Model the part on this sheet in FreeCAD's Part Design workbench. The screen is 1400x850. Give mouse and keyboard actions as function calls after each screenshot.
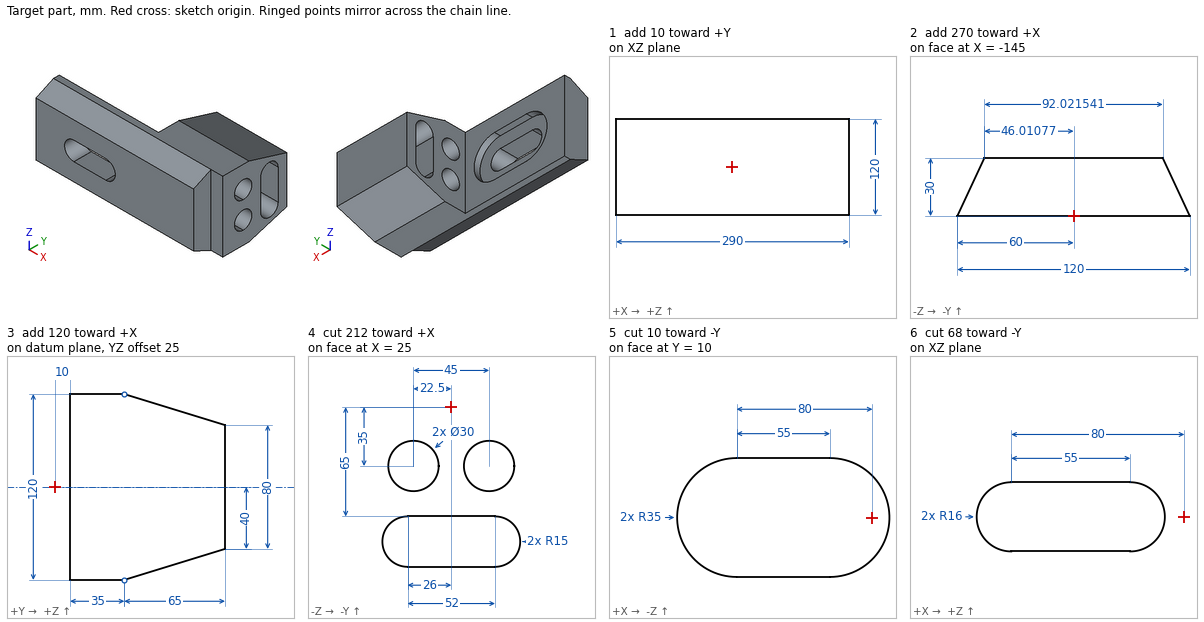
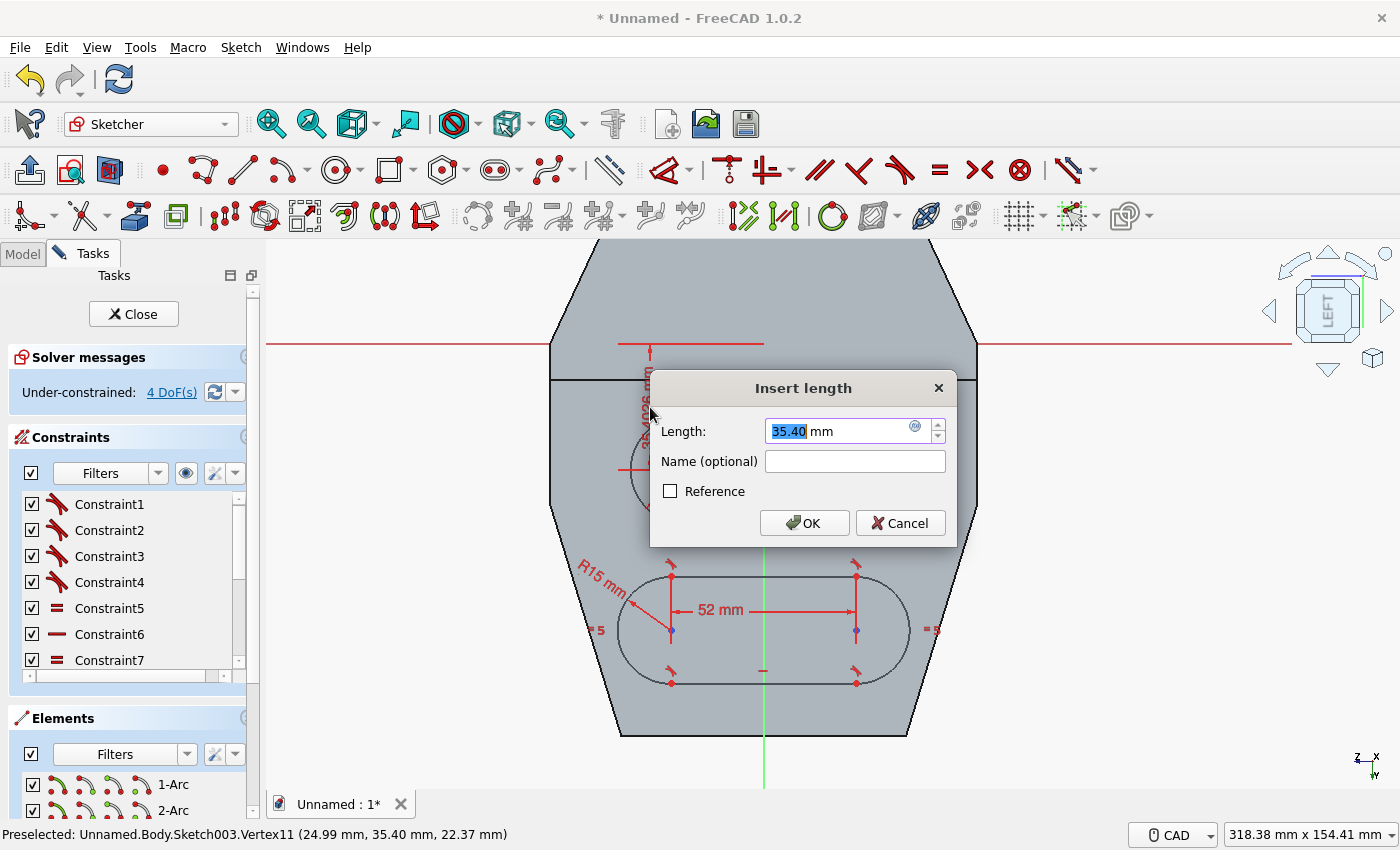
text(35)
key(Return)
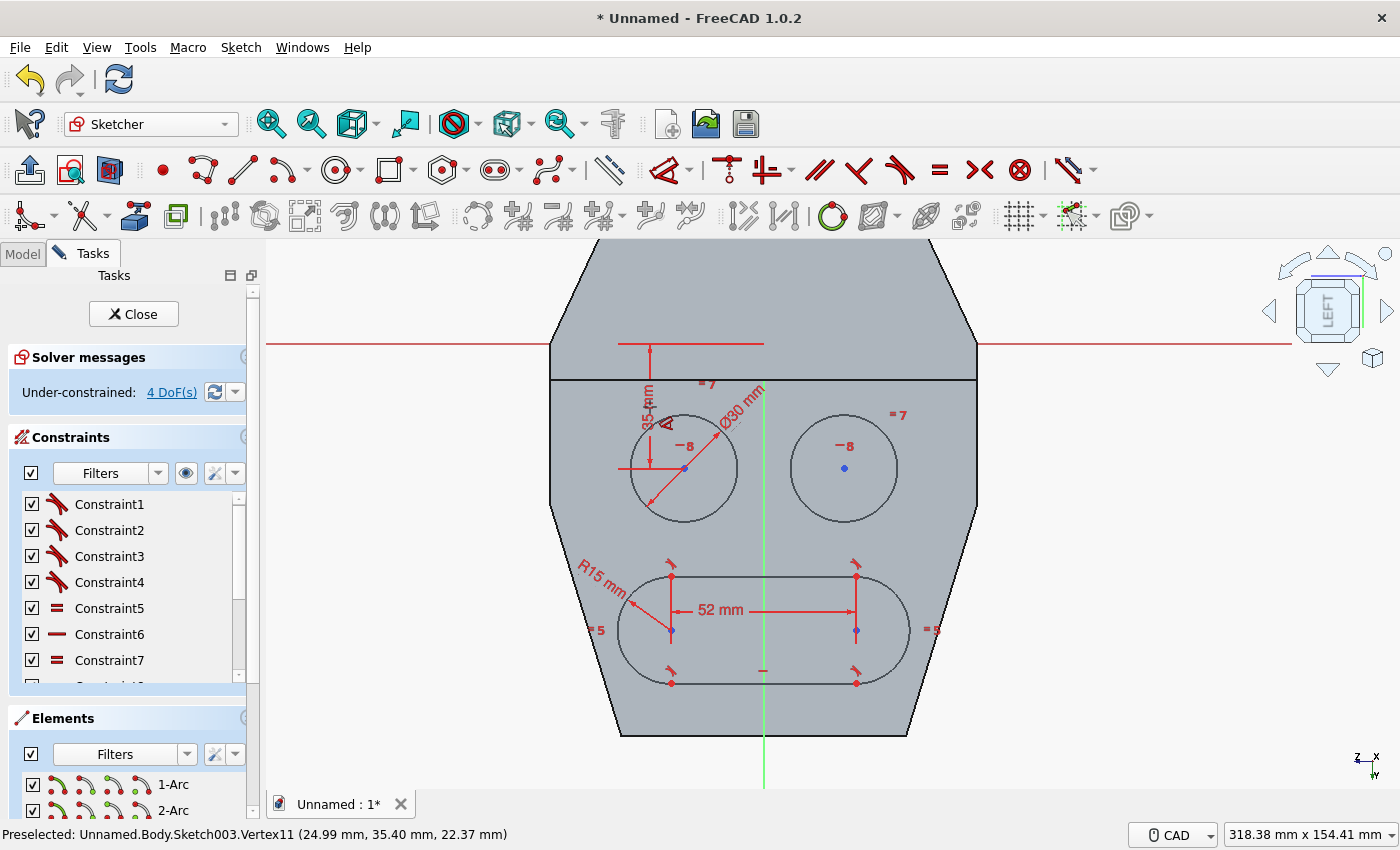
click(671, 577)
click(717, 310)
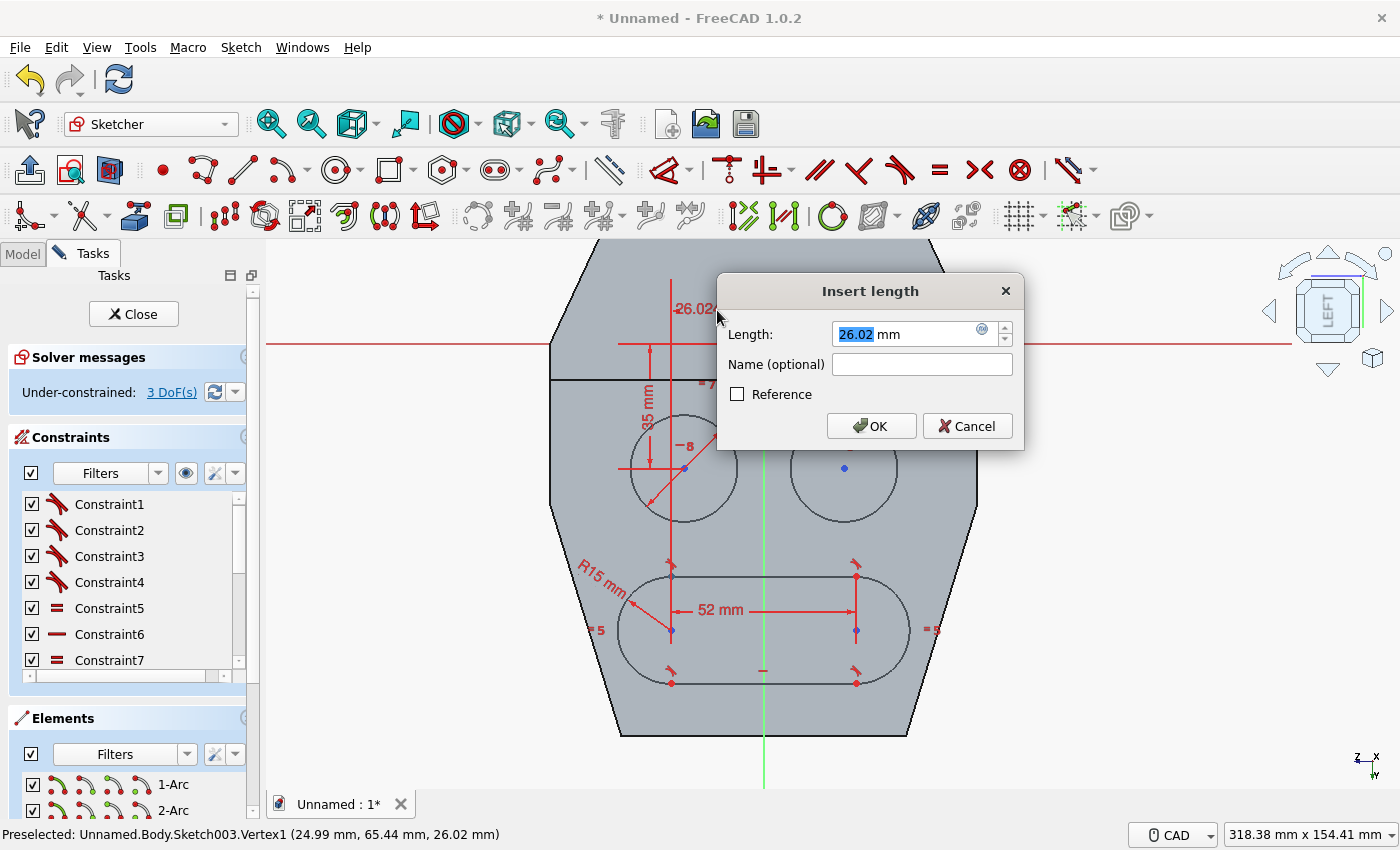
text(26)
key(Return)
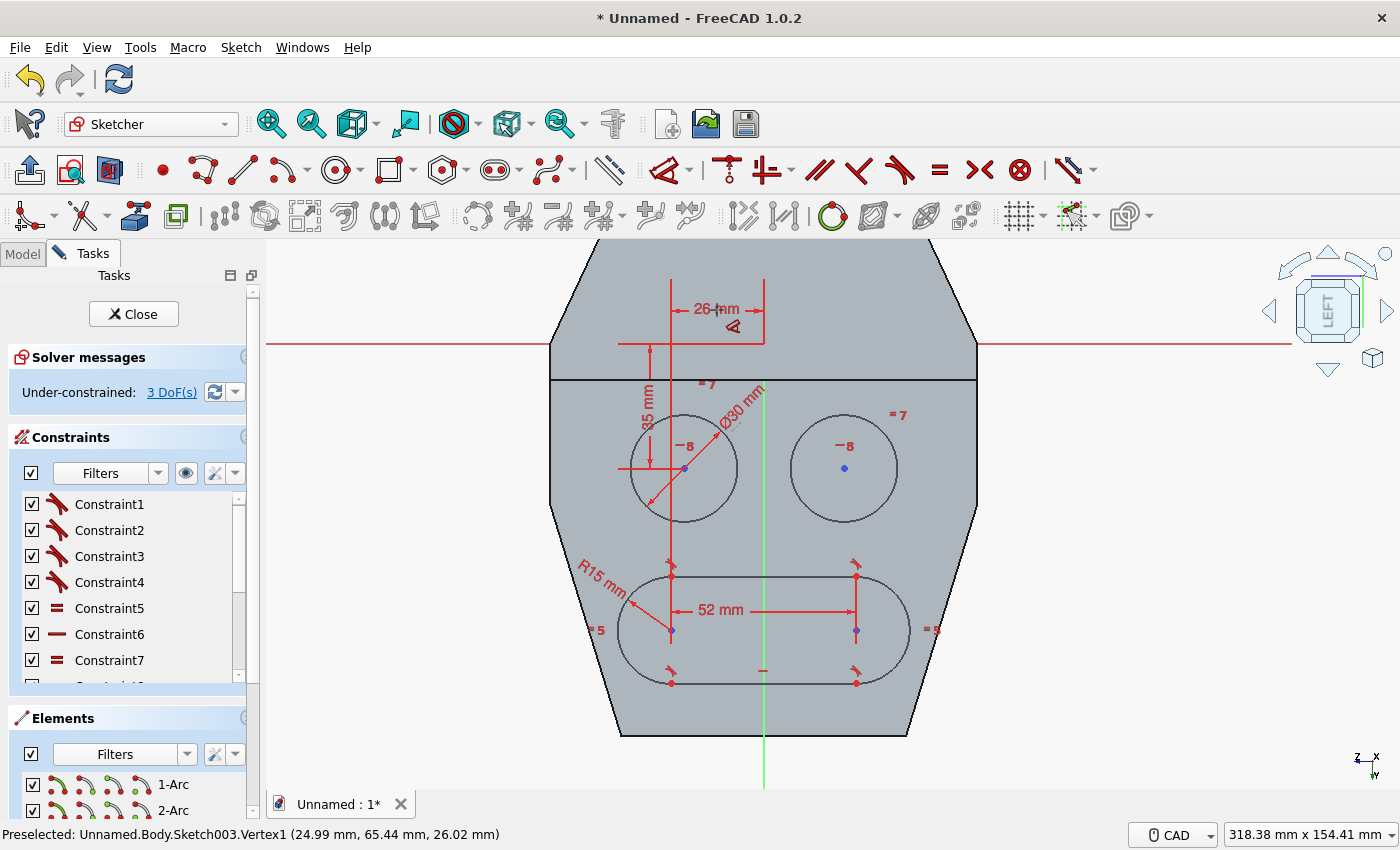
click(671, 577)
click(637, 379)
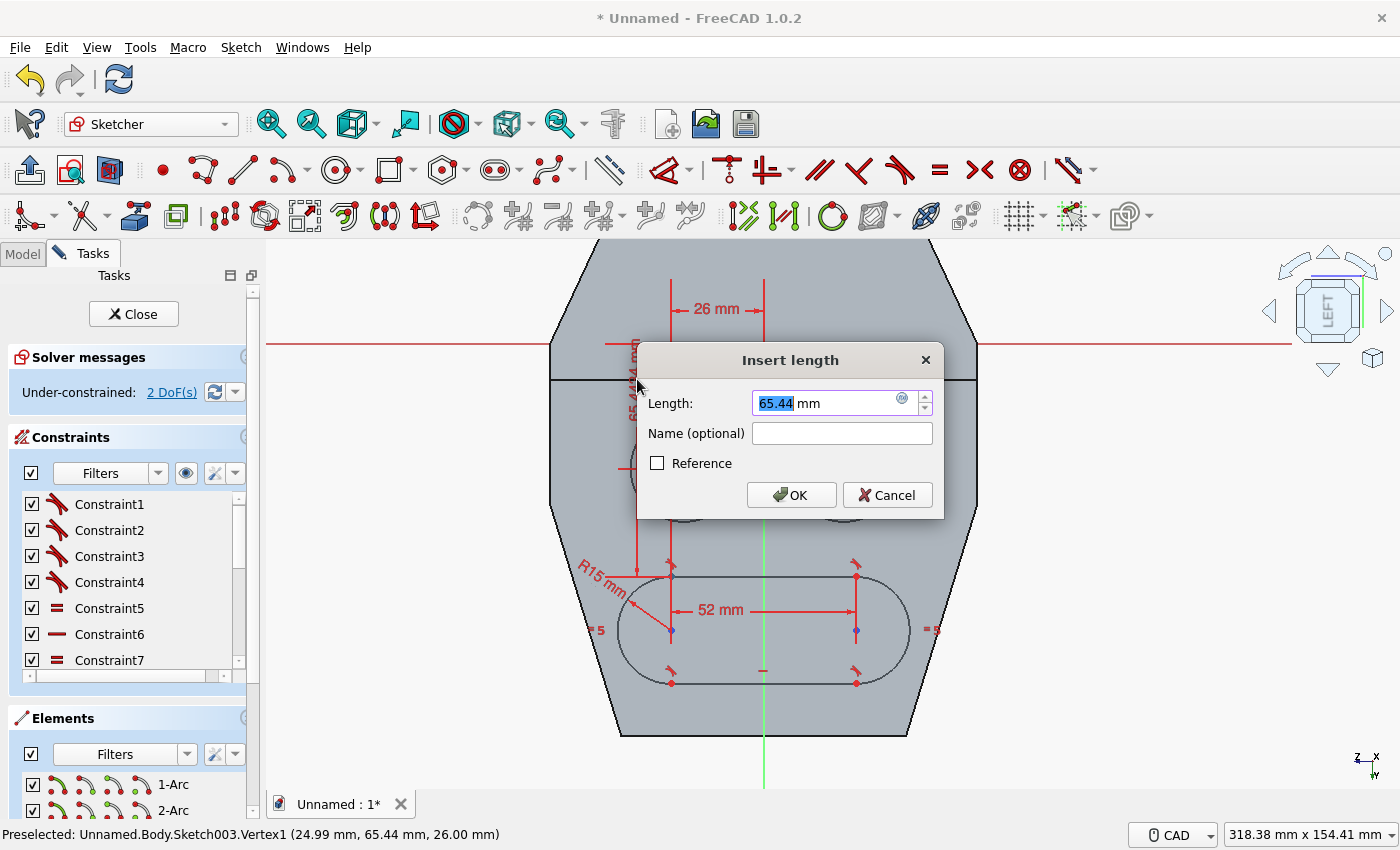
text(65)
key(Return)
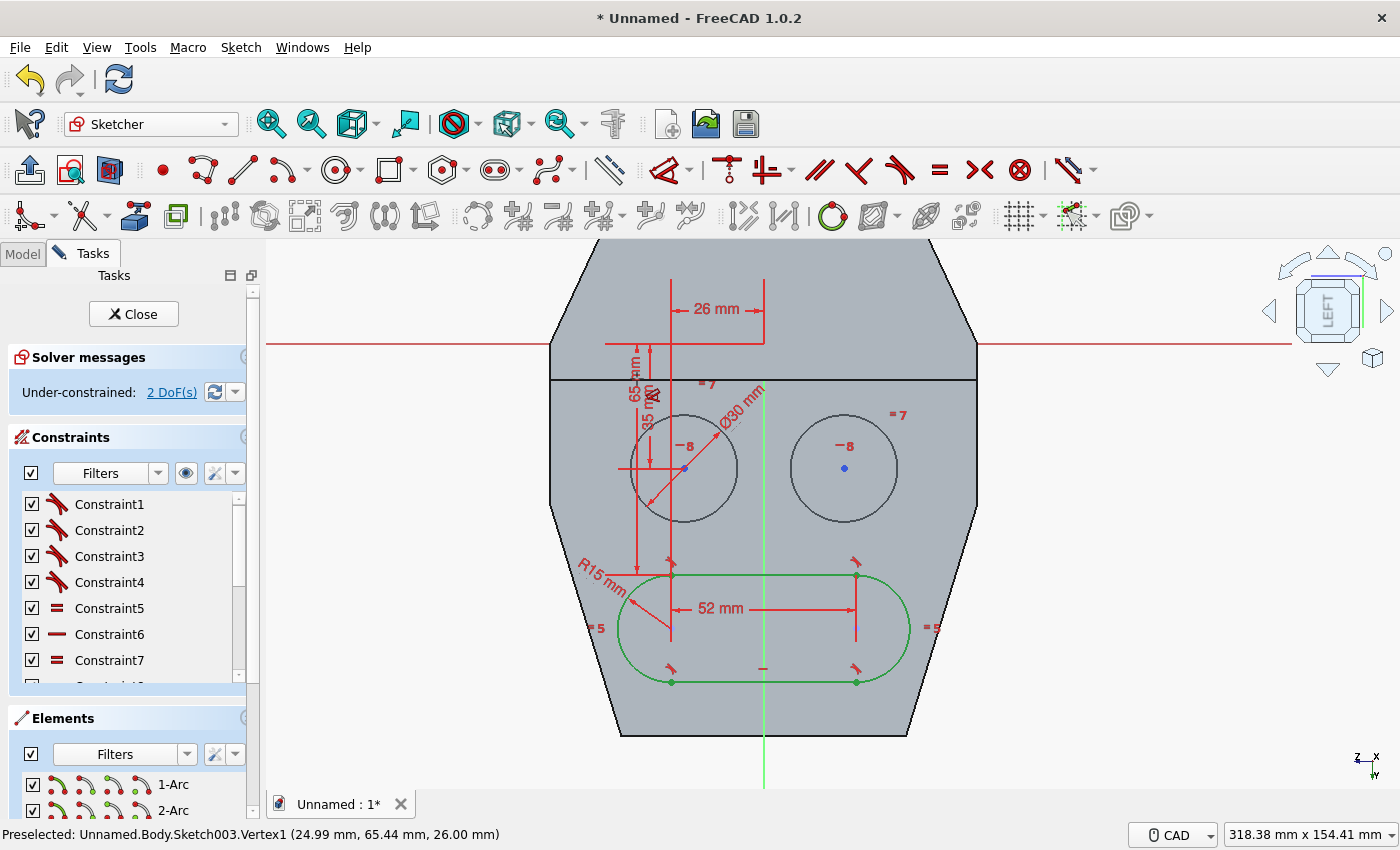
click(684, 469)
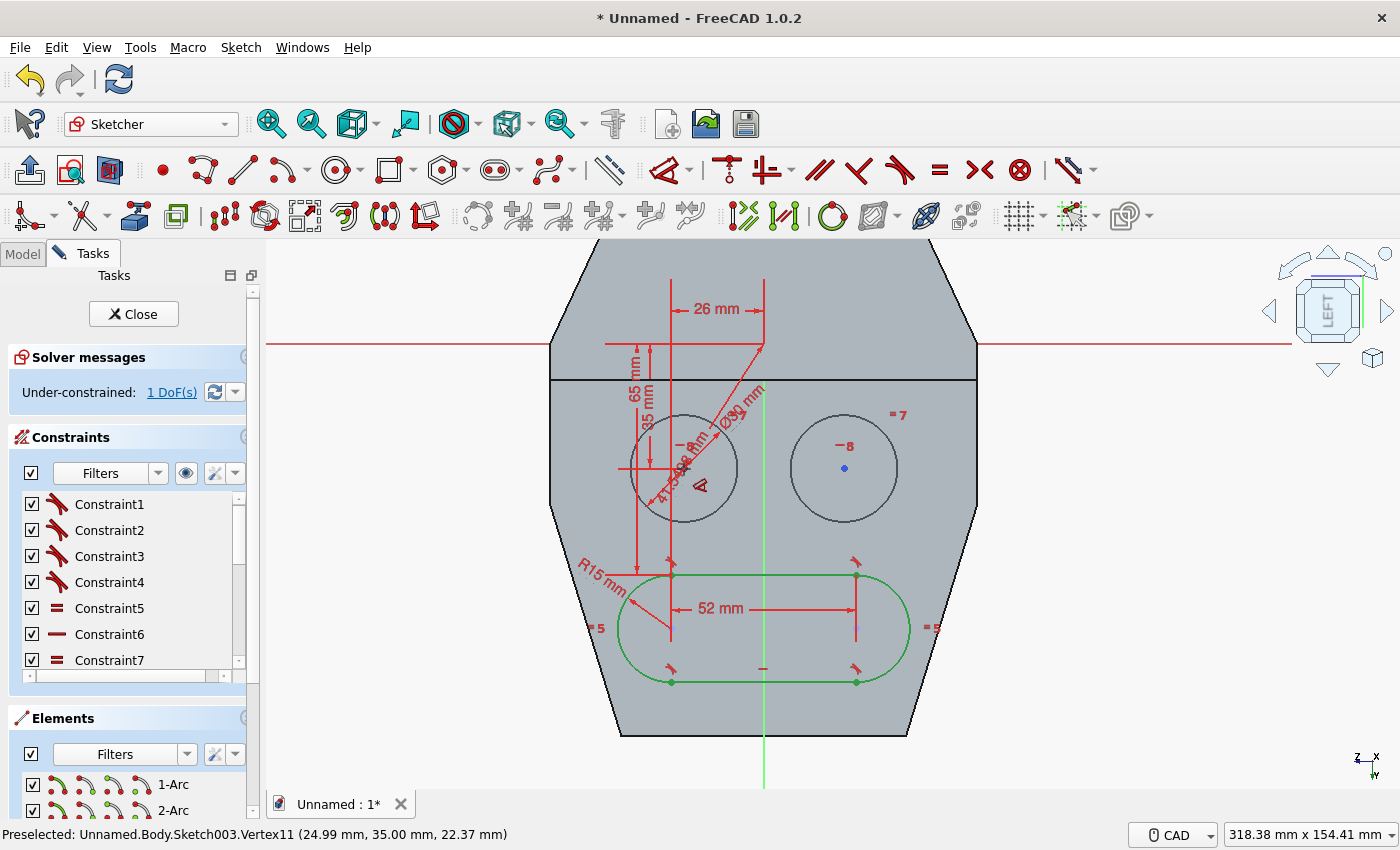
click(844, 469)
click(727, 527)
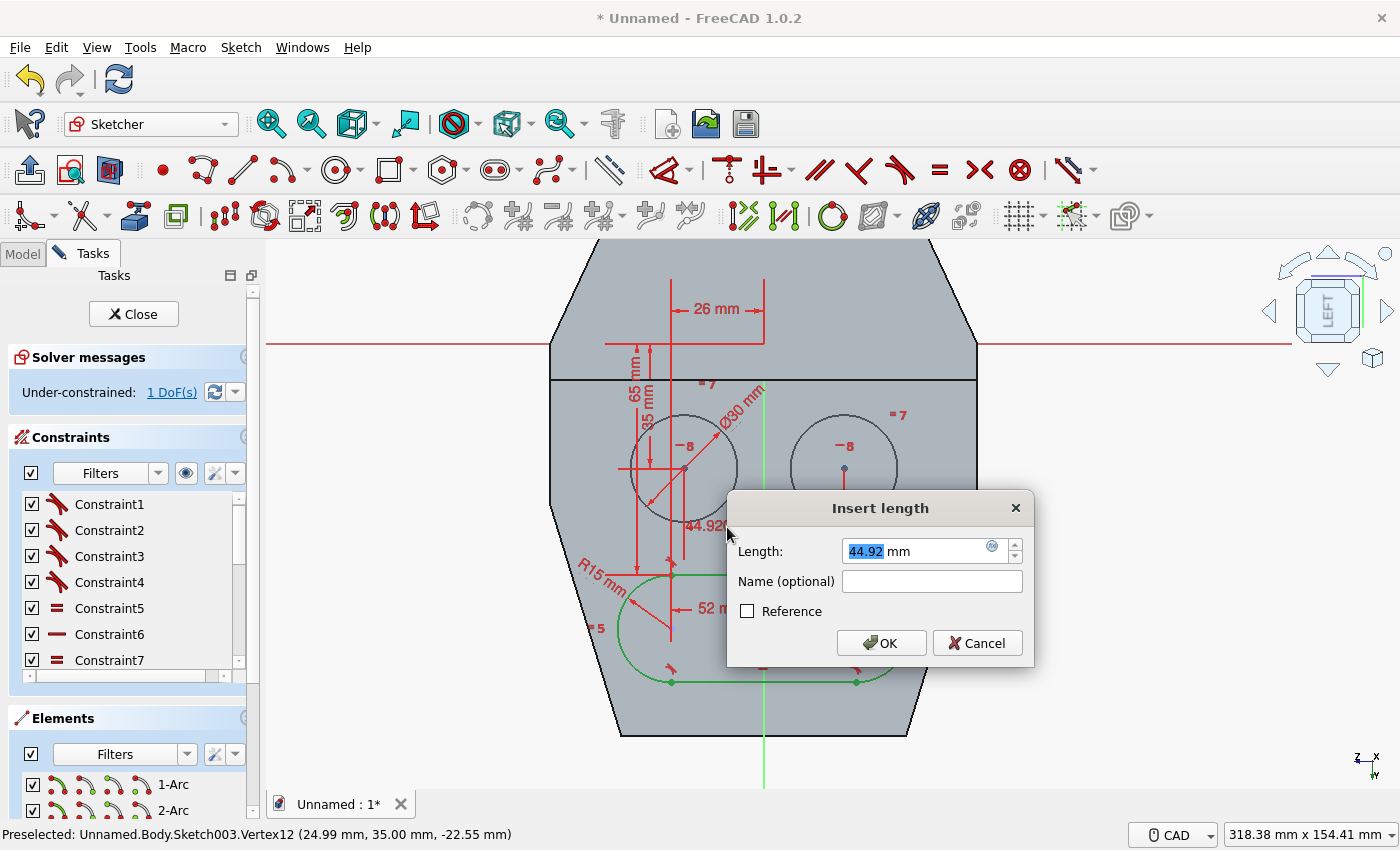
text(45)
key(Return)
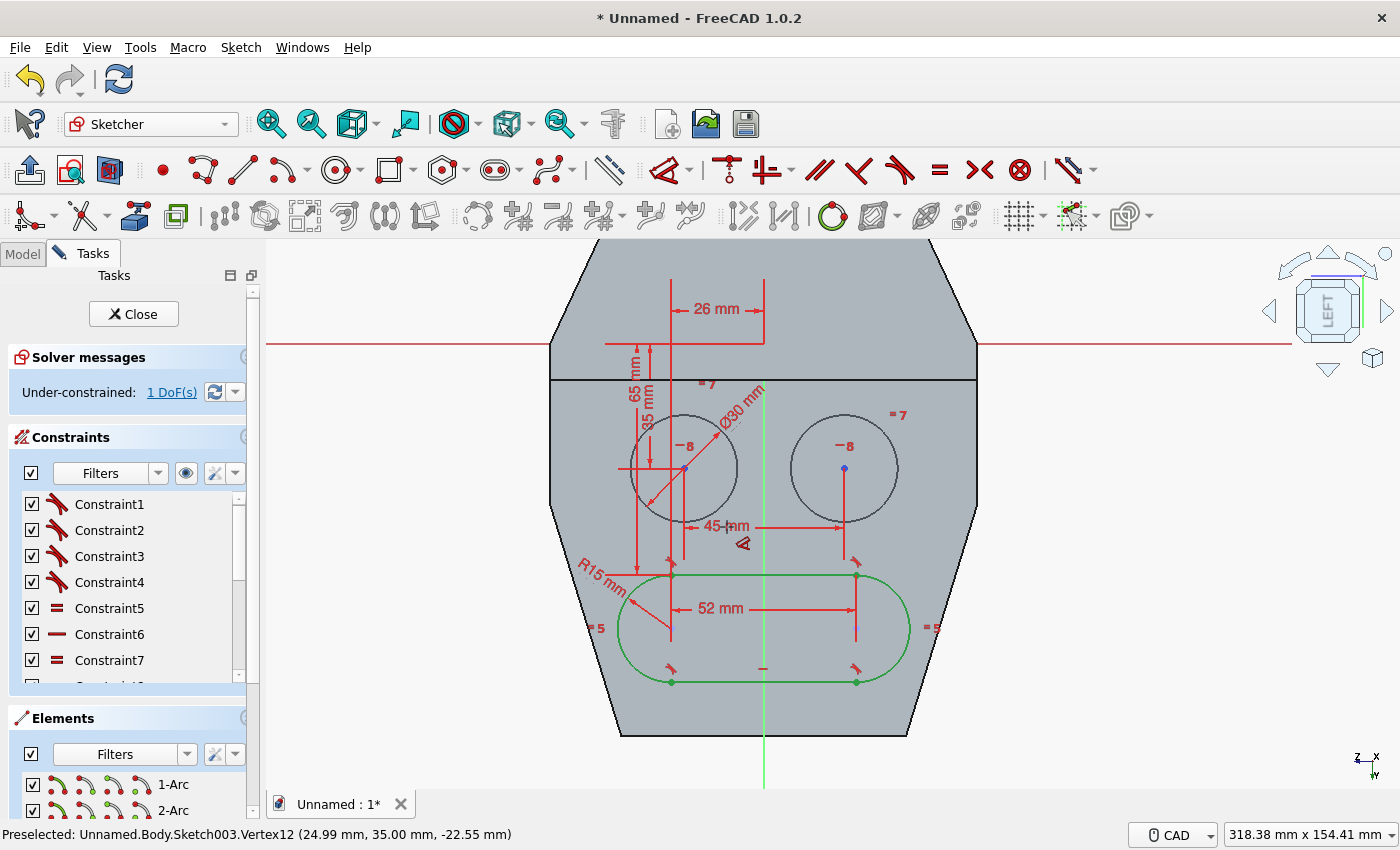
click(684, 469)
click(706, 503)